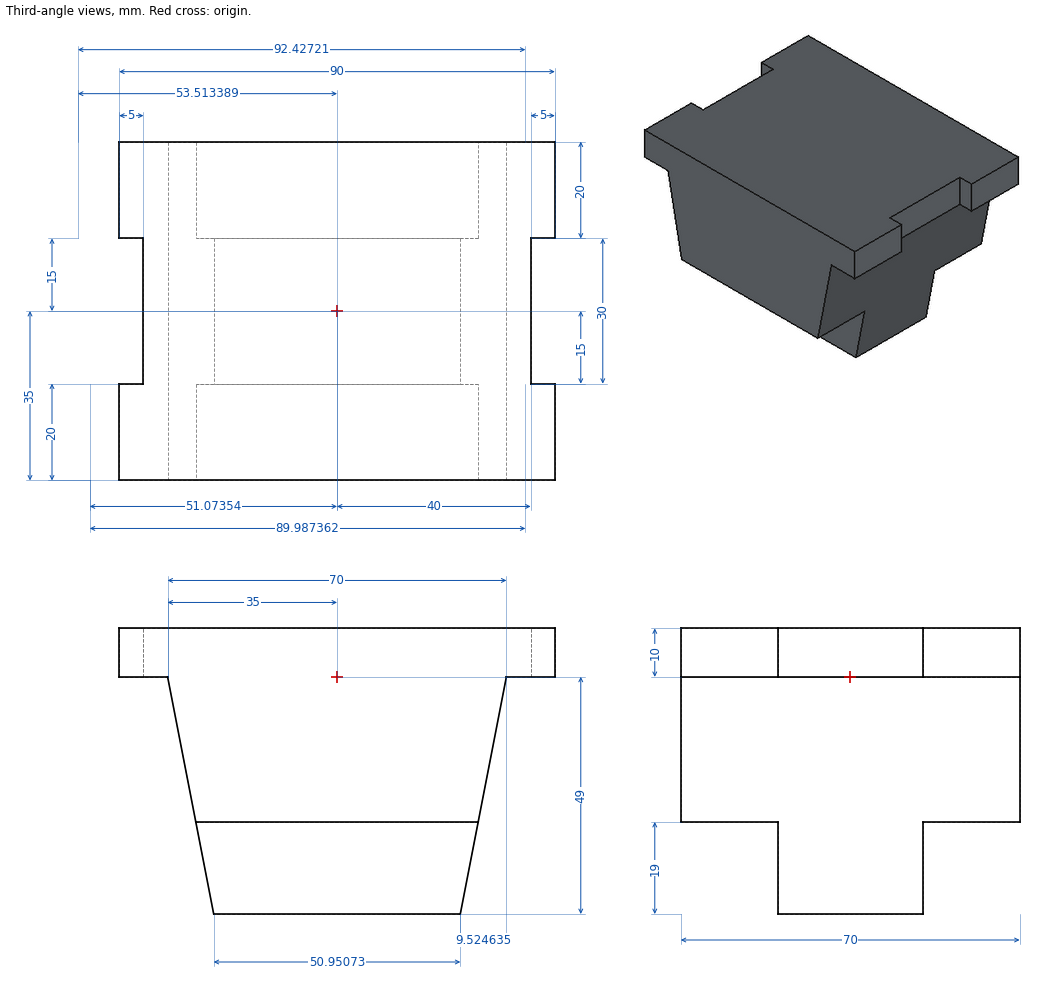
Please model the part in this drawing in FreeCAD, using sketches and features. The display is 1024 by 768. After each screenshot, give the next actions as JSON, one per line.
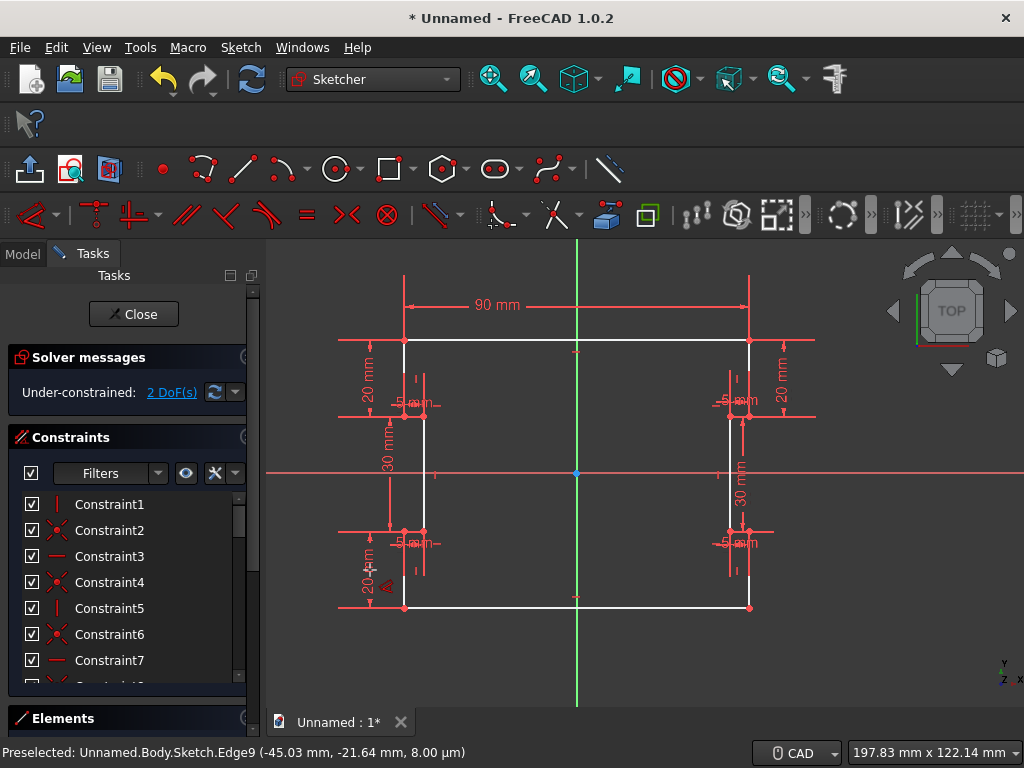
{"action": "left_click", "coordinate": [730, 532]}
{"action": "left_click", "coordinate": [654, 566]}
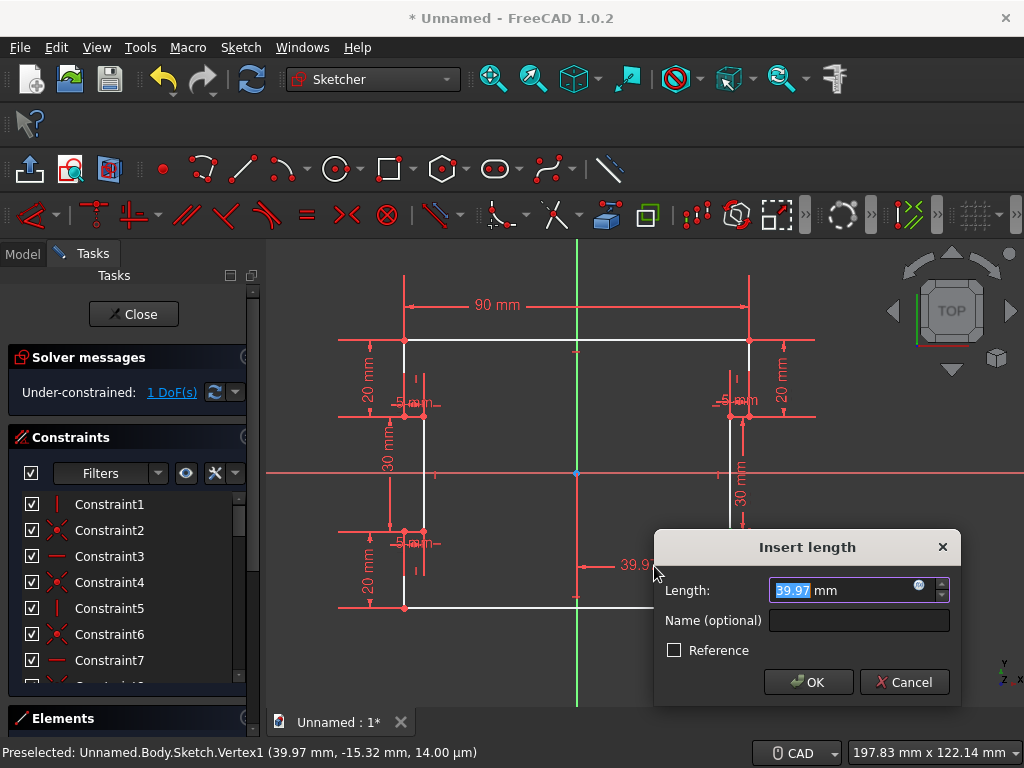
{"action": "type", "text": "40"}
{"action": "key", "text": "Return"}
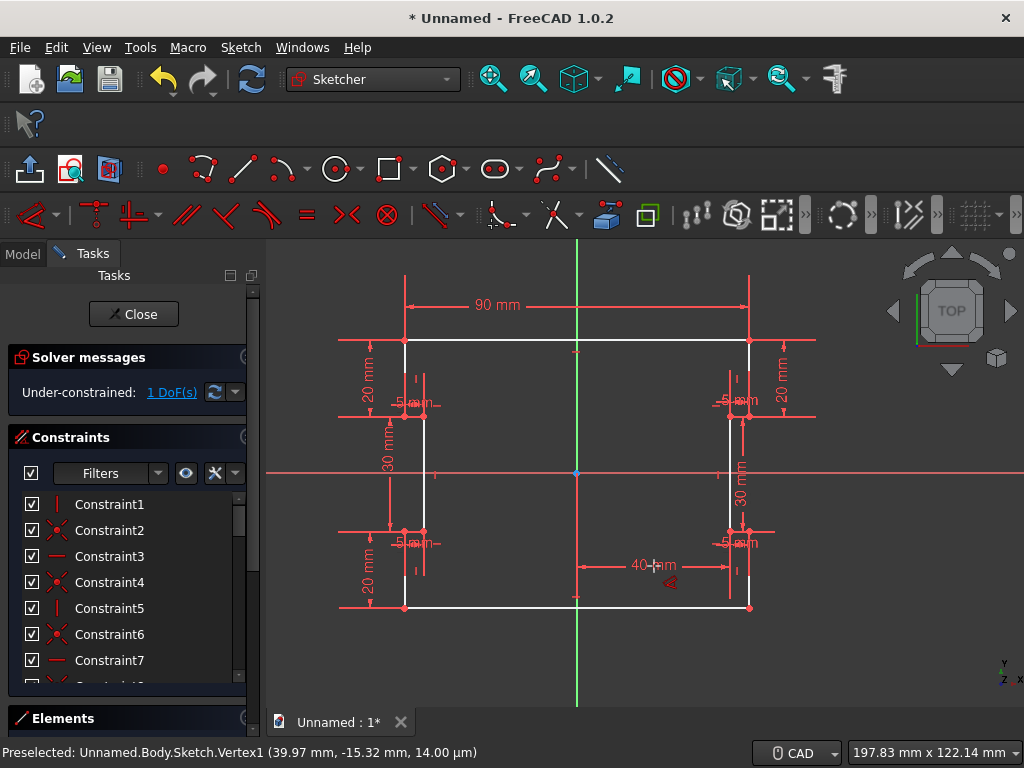
{"action": "left_click", "coordinate": [730, 532]}
{"action": "left_click", "coordinate": [764, 516]}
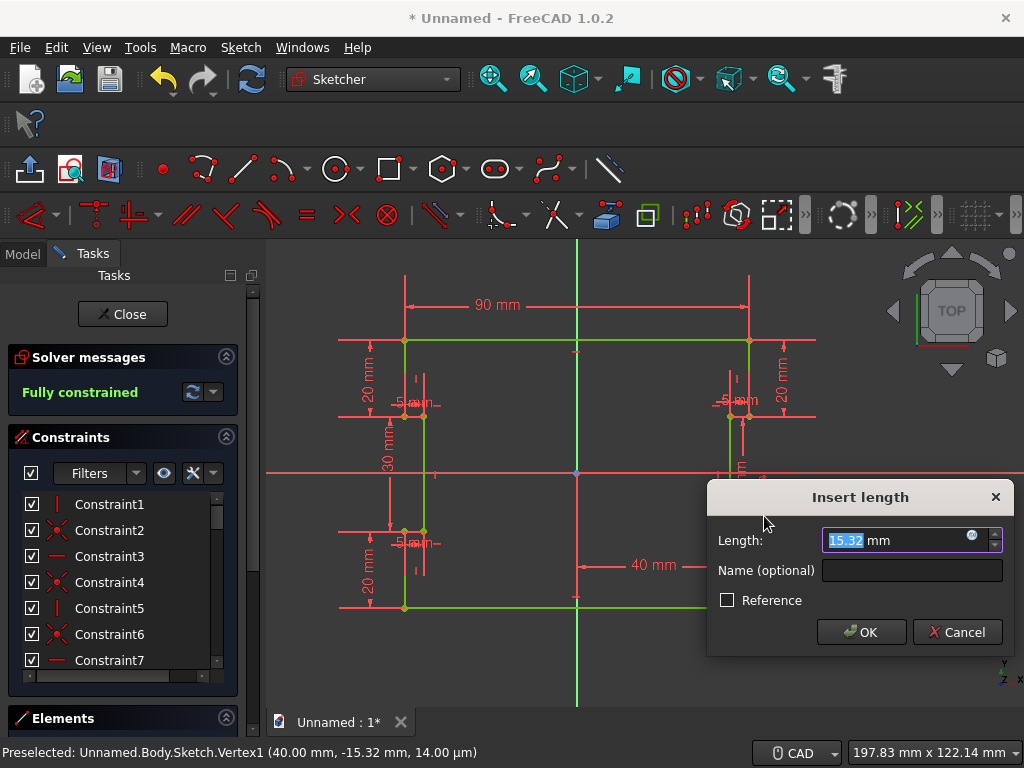
{"action": "type", "text": "15"}
{"action": "key", "text": "Return"}
{"action": "key", "text": "Escape"}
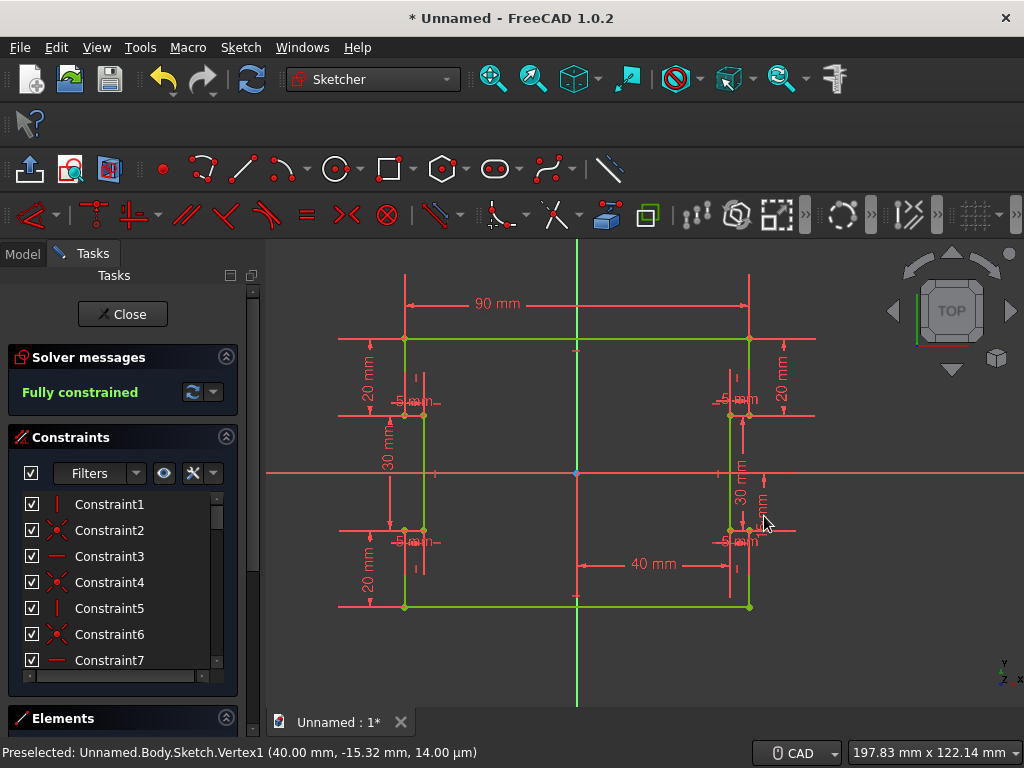
{"action": "left_click", "coordinate": [123, 314]}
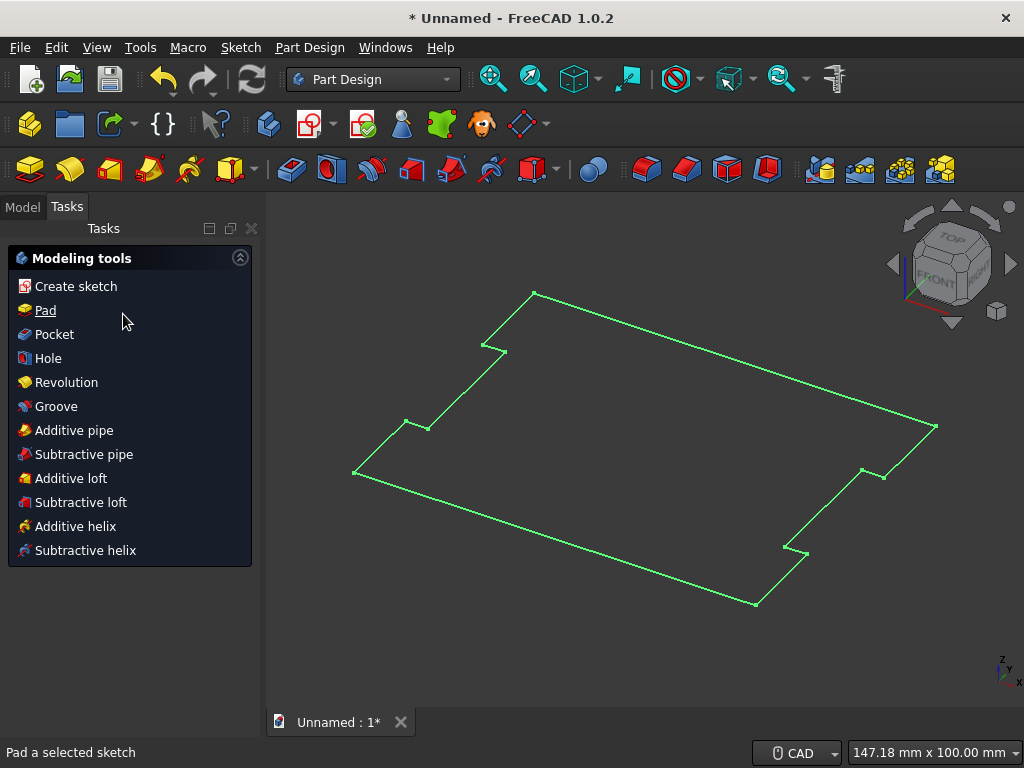
{"action": "left_click", "coordinate": [30, 170]}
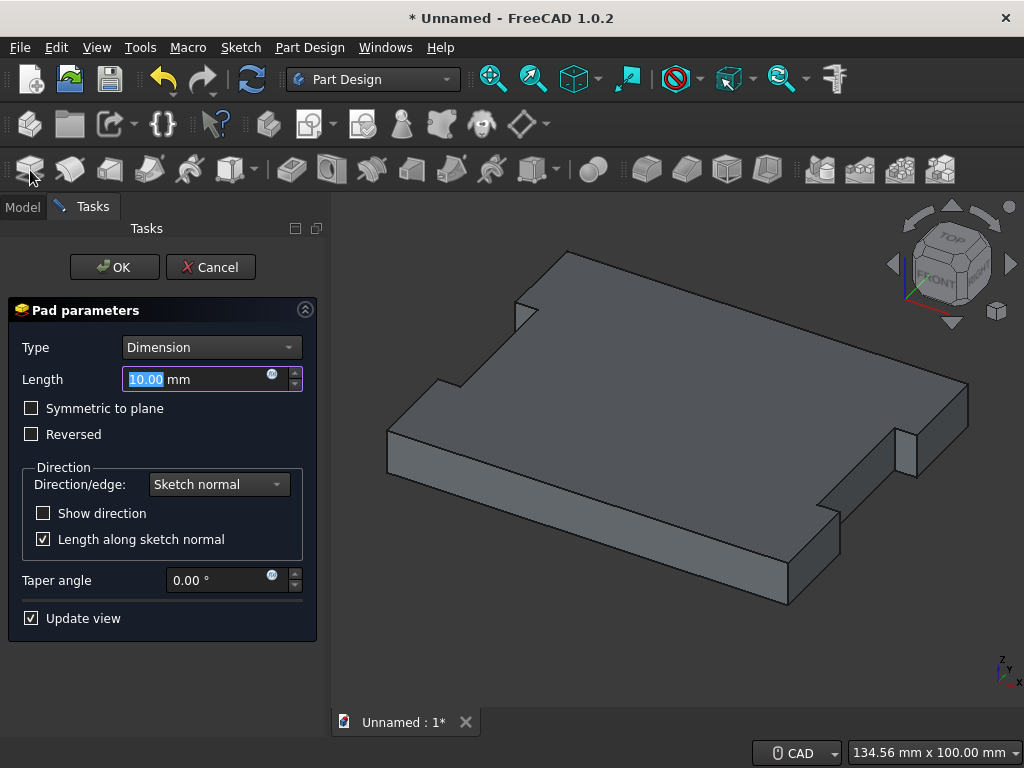
{"action": "type", "text": "10"}
{"action": "key", "text": "Tab"}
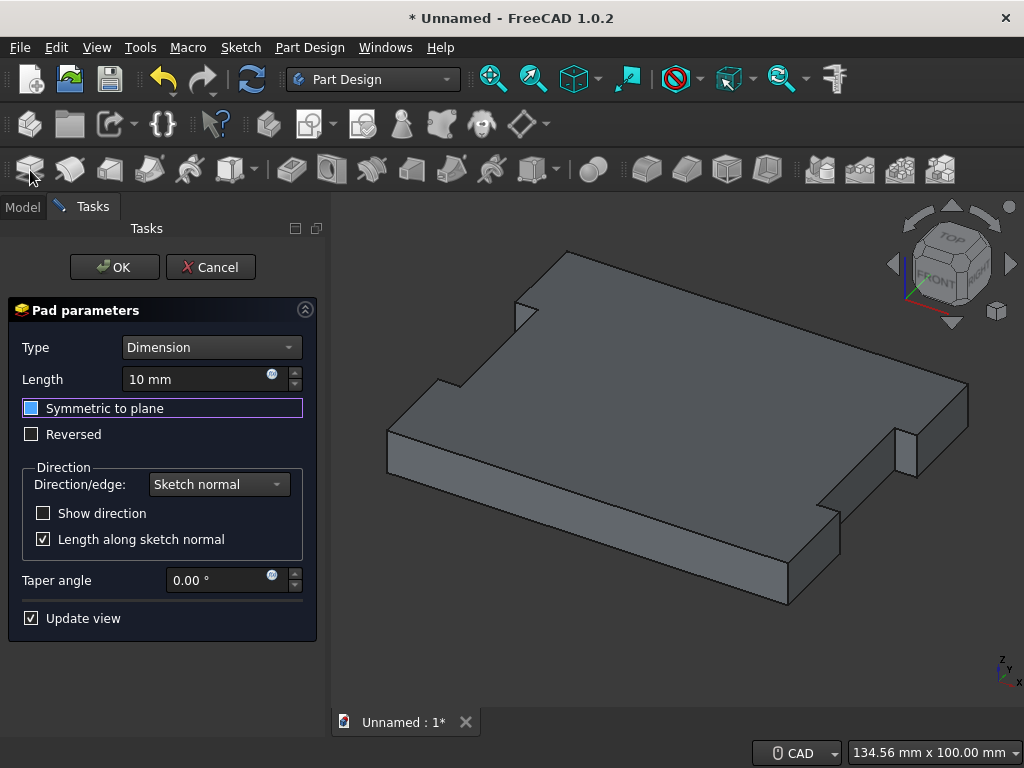
{"action": "left_click", "coordinate": [115, 267]}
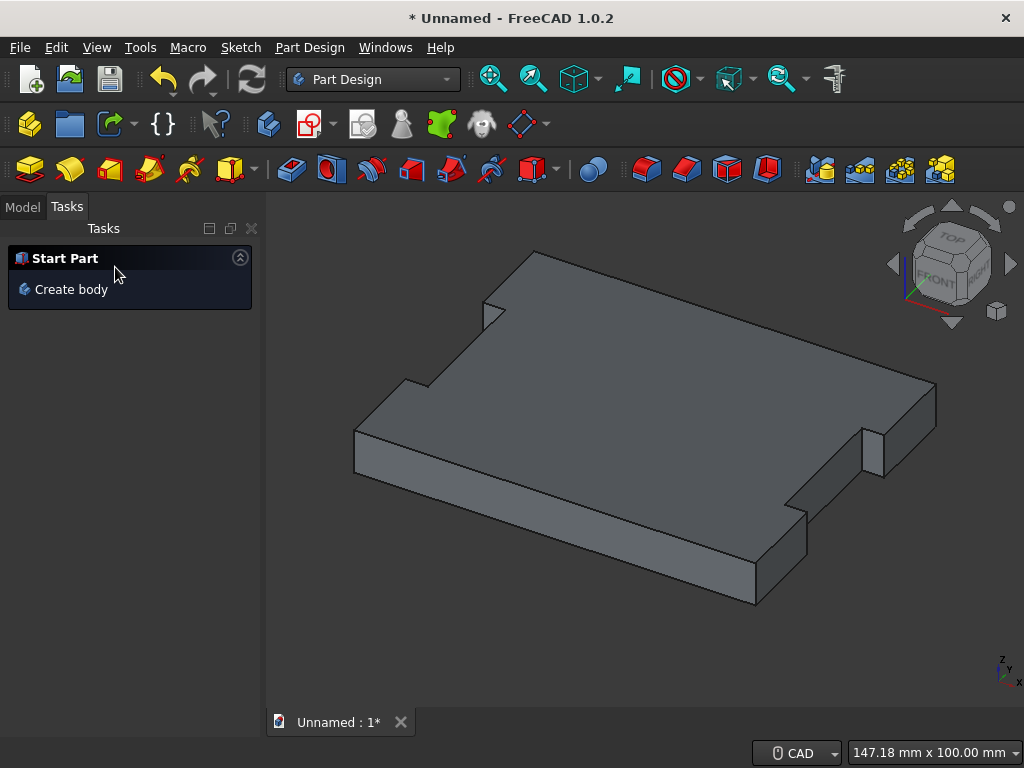
{"action": "key", "text": "4"}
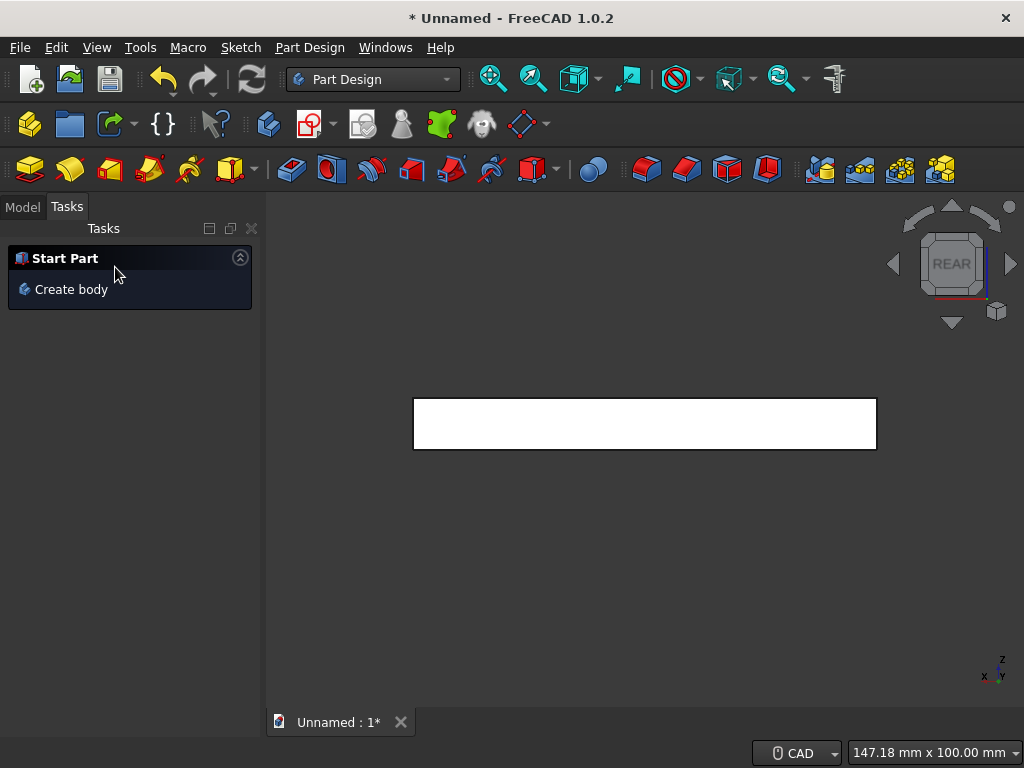
{"action": "left_click", "coordinate": [446, 423]}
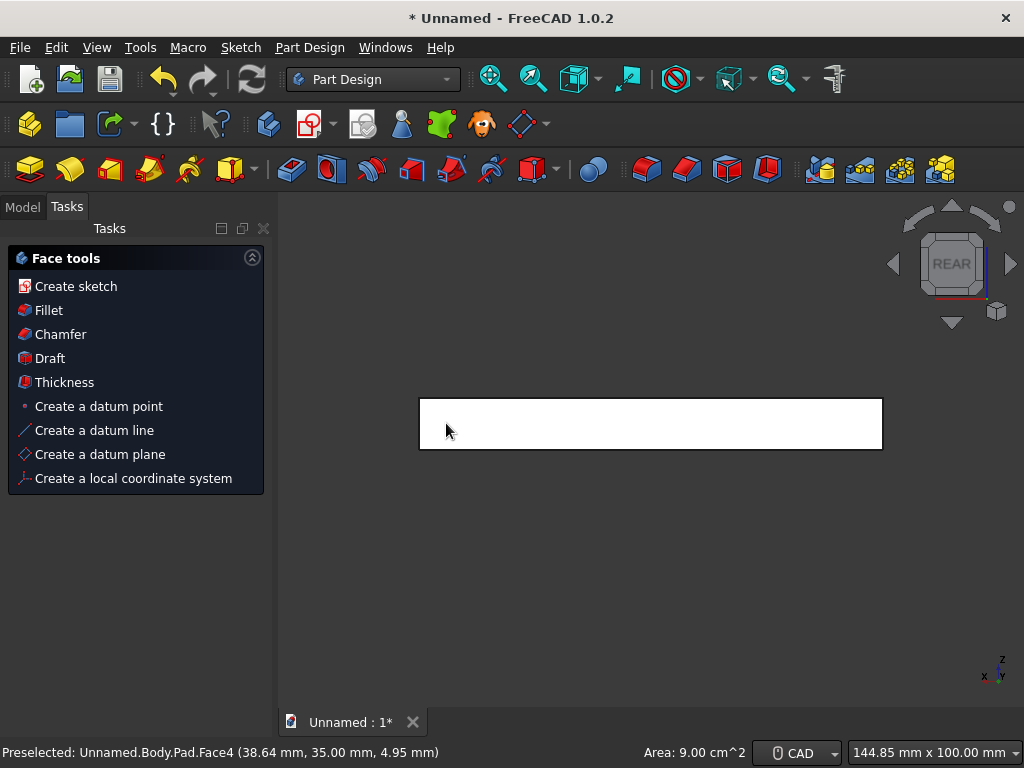
{"action": "left_click", "coordinate": [310, 124]}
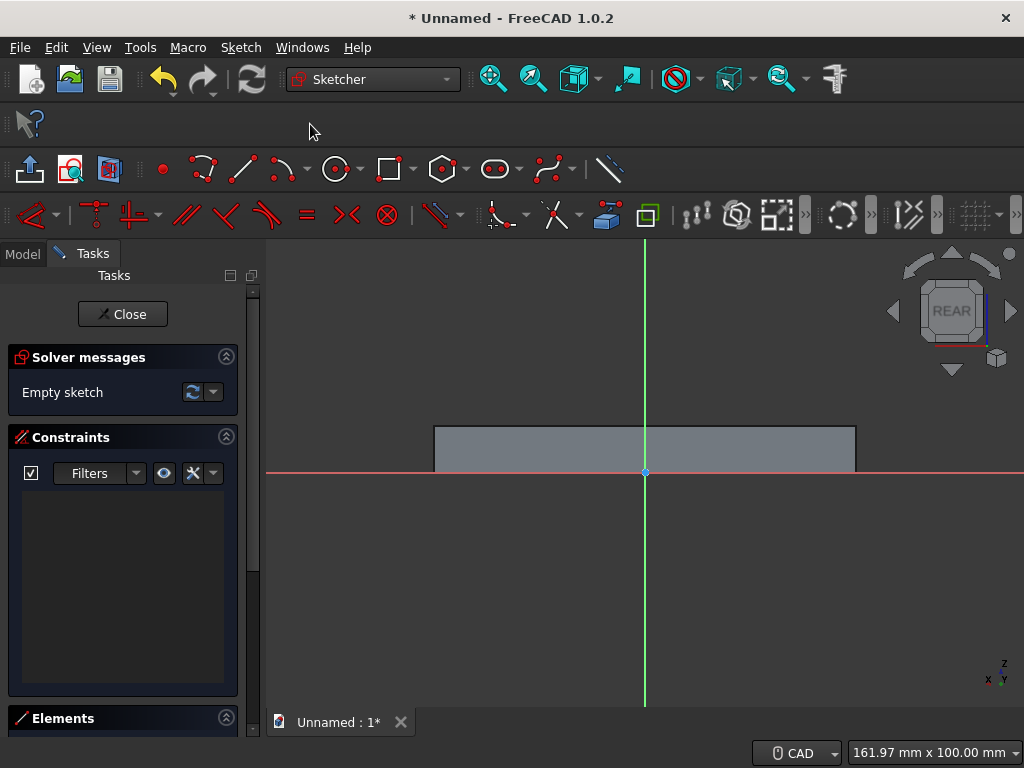
{"action": "scroll", "coordinate": [294, 267], "scroll_direction": "down", "scroll_amount": 1}